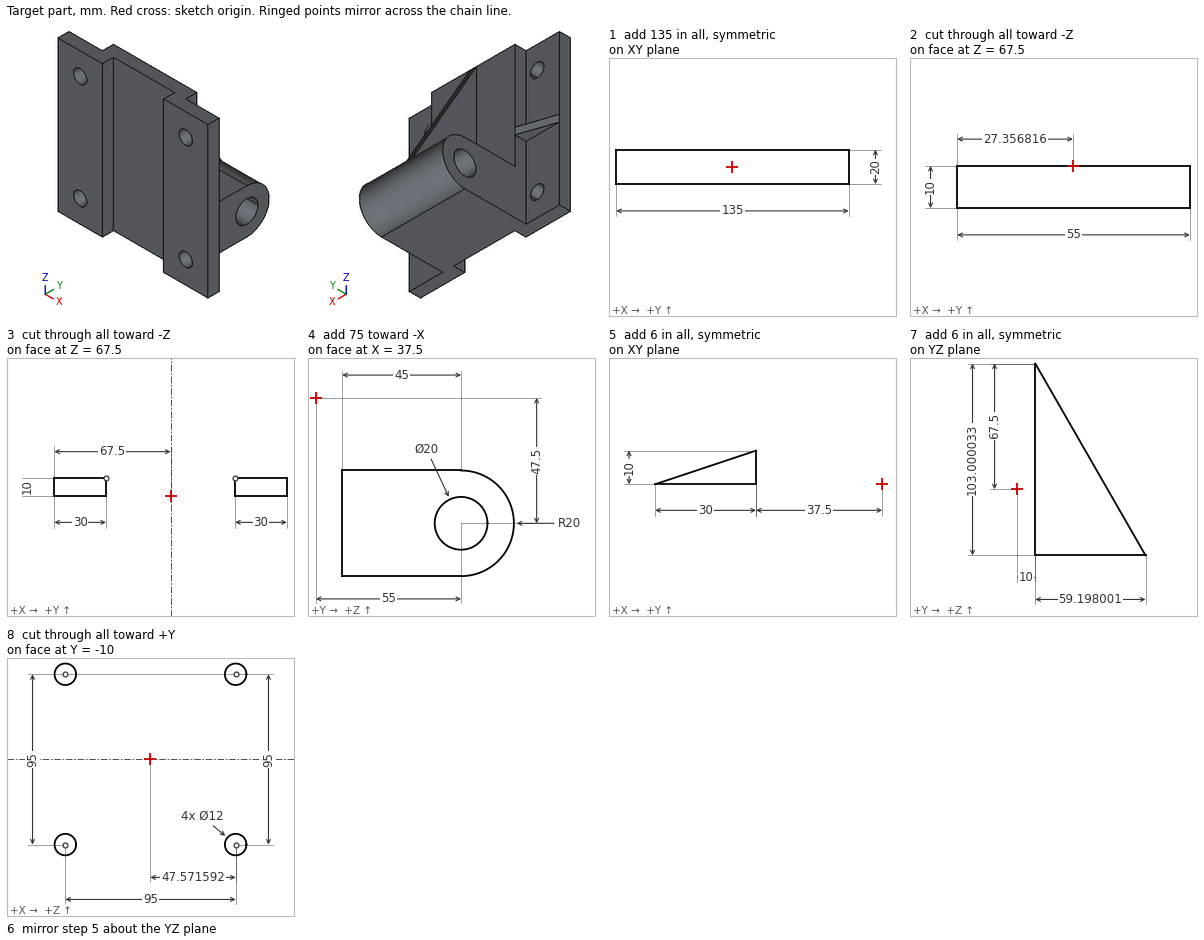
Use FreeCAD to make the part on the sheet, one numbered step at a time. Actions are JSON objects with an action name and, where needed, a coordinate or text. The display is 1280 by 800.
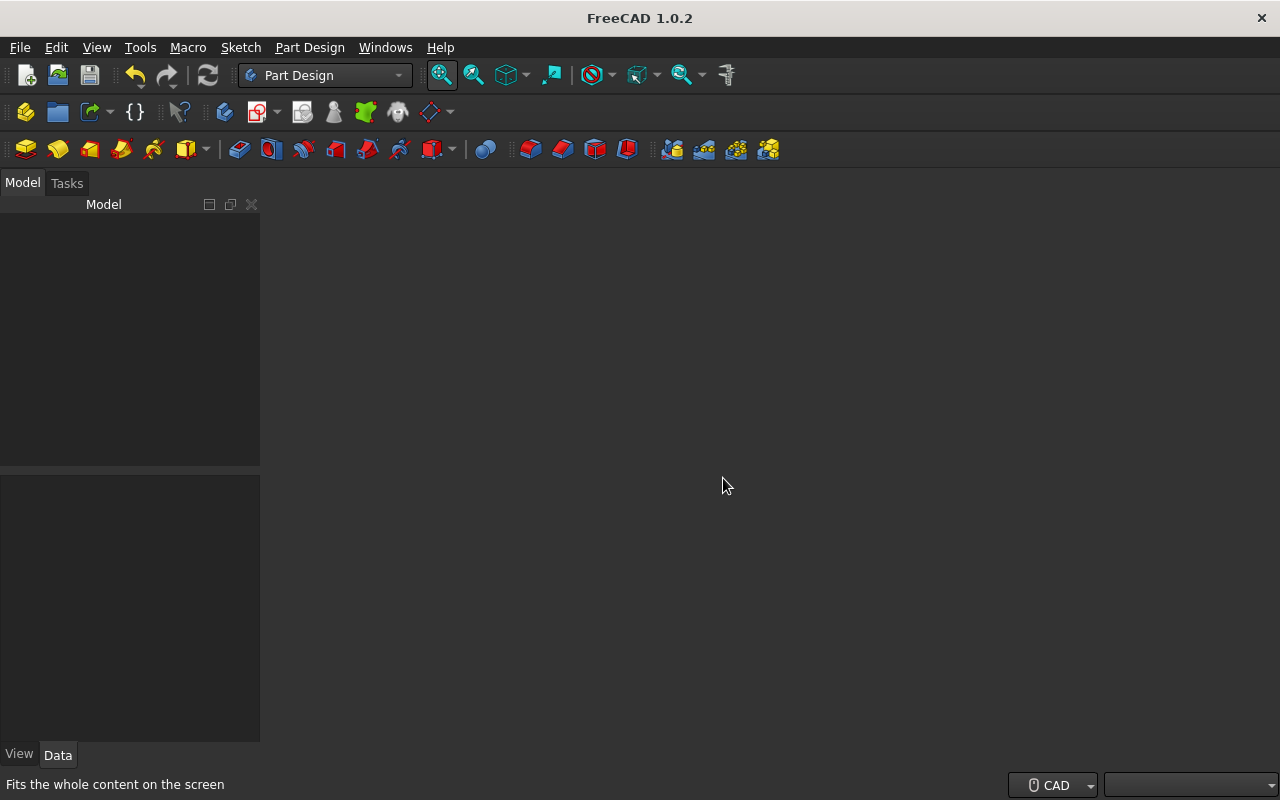
{"action": "left_click", "coordinate": [26, 76]}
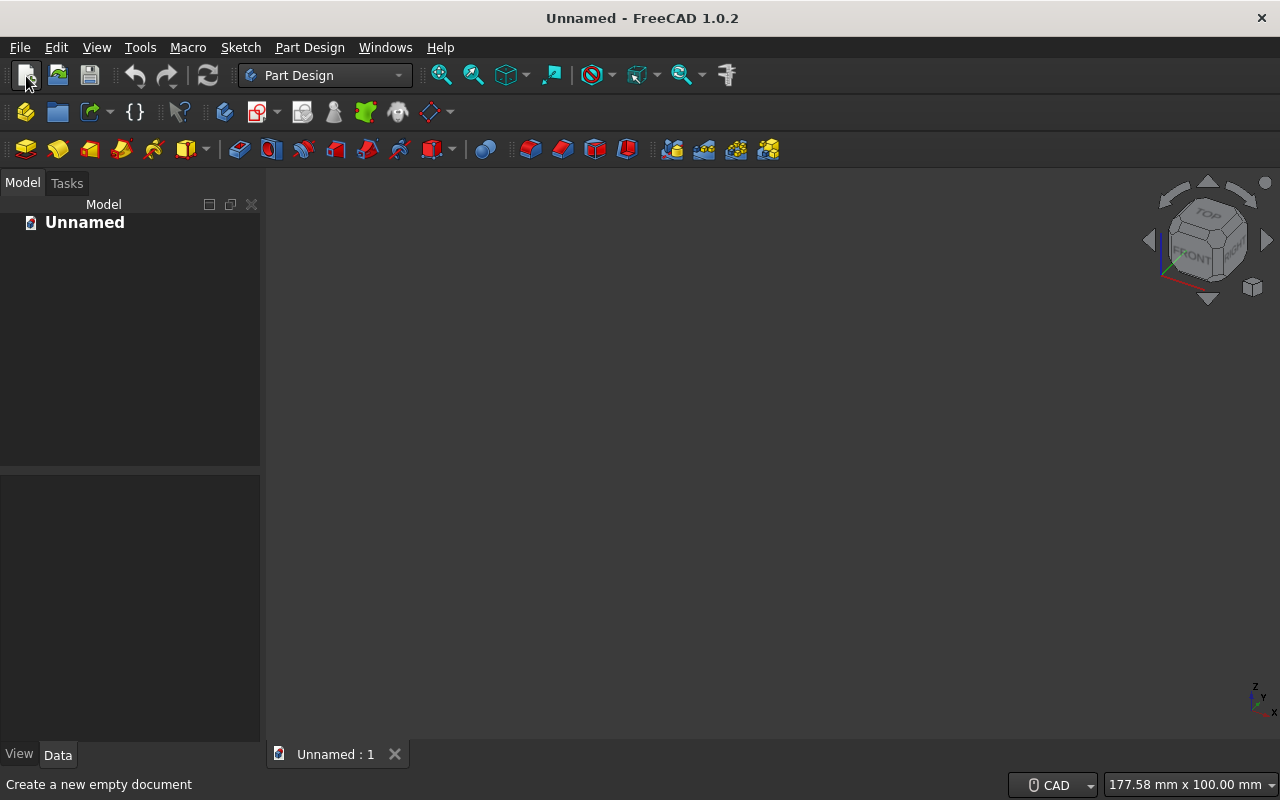
{"action": "left_click", "coordinate": [258, 112]}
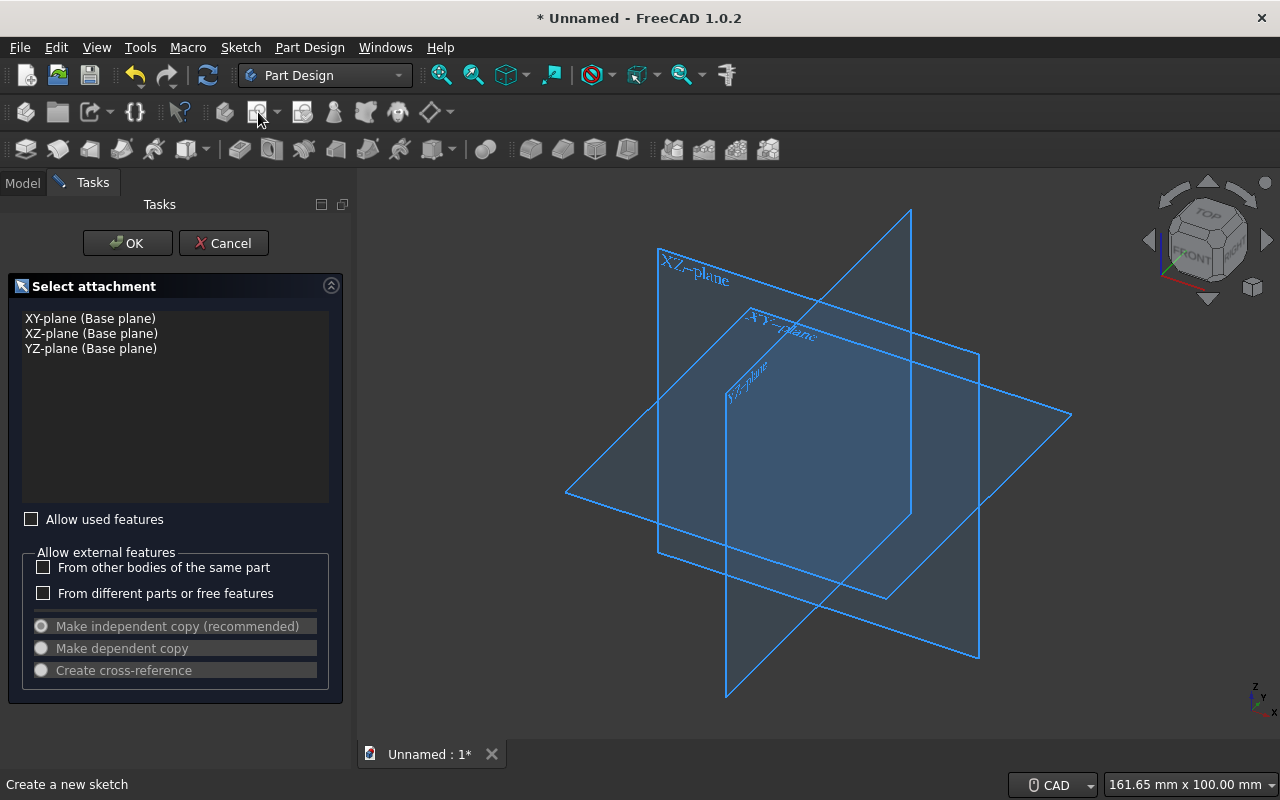
{"action": "left_click", "coordinate": [82, 318]}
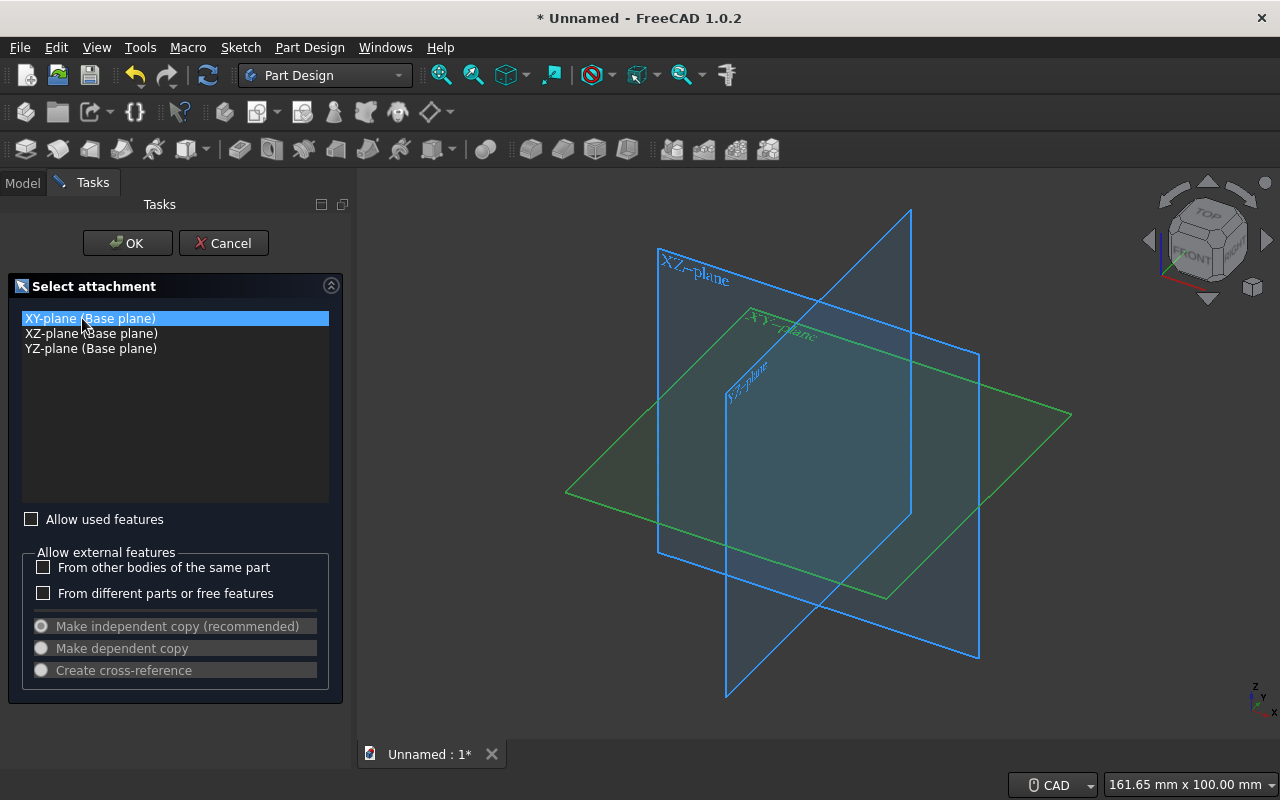
{"action": "left_click", "coordinate": [128, 243]}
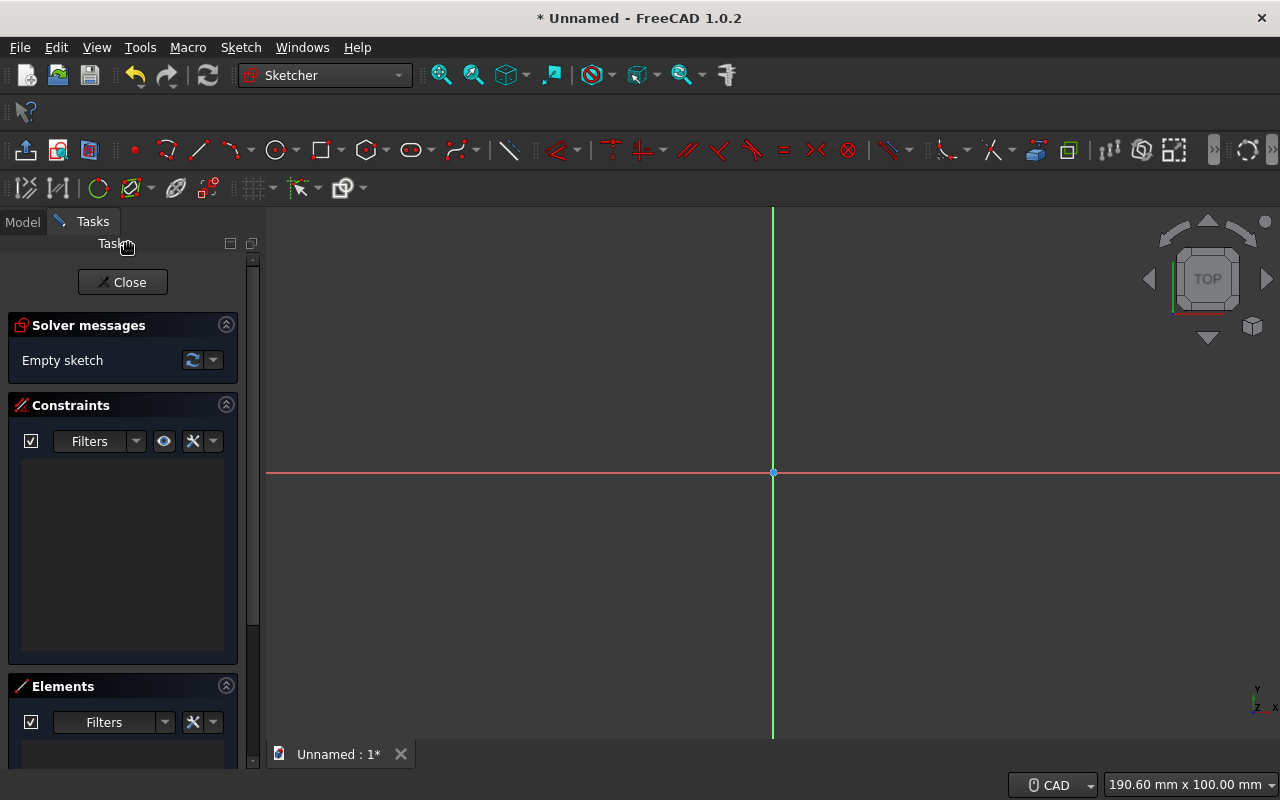
{"action": "scroll", "coordinate": [395, 473], "scroll_direction": "down", "scroll_amount": 1}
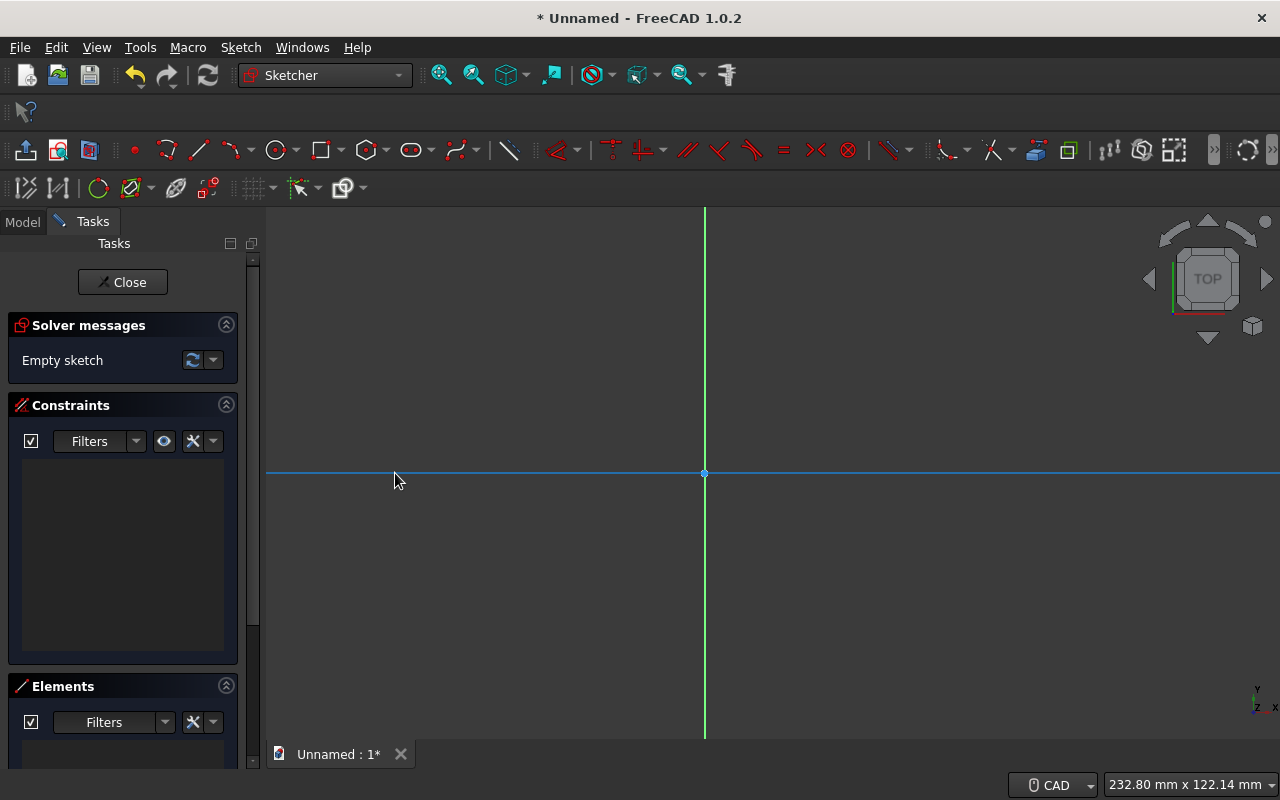
{"action": "key", "text": "g v"}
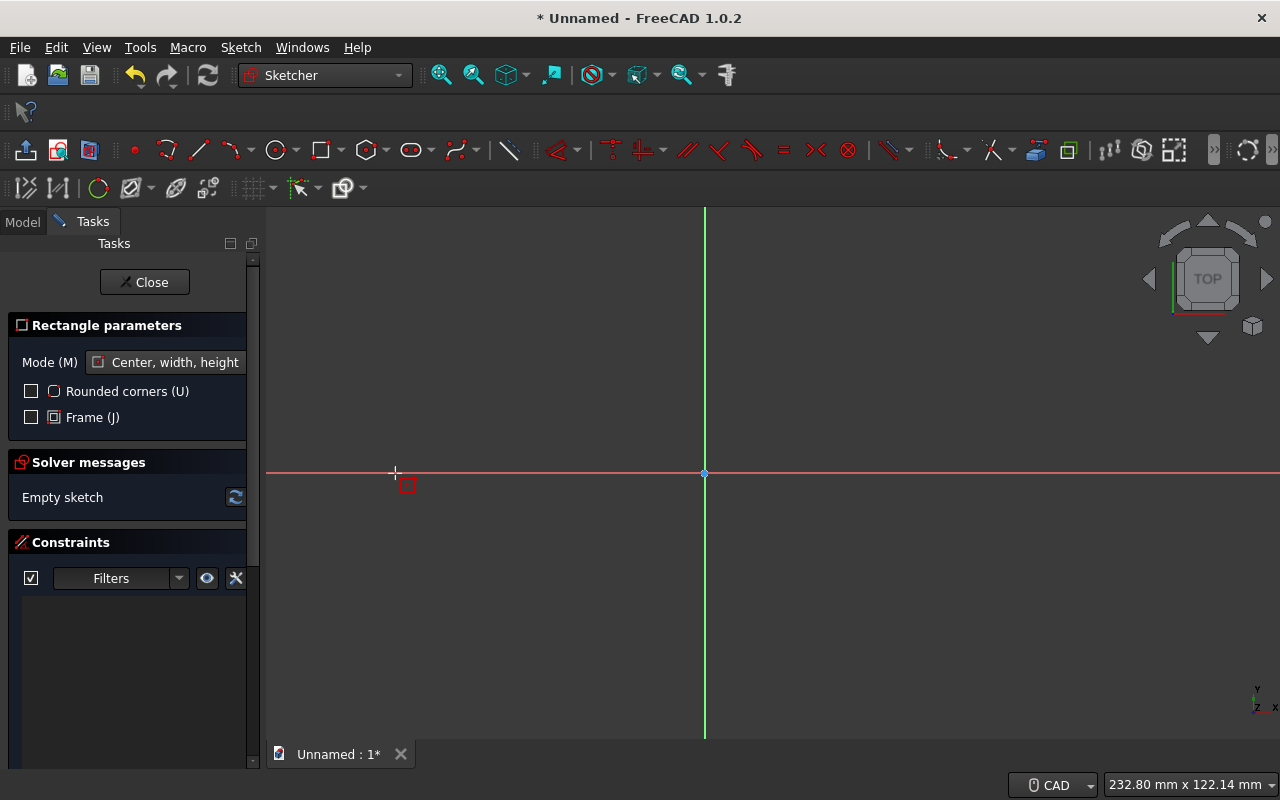
{"action": "left_click", "coordinate": [705, 473]}
{"action": "left_click", "coordinate": [999, 430]}
{"action": "key", "text": "Escape"}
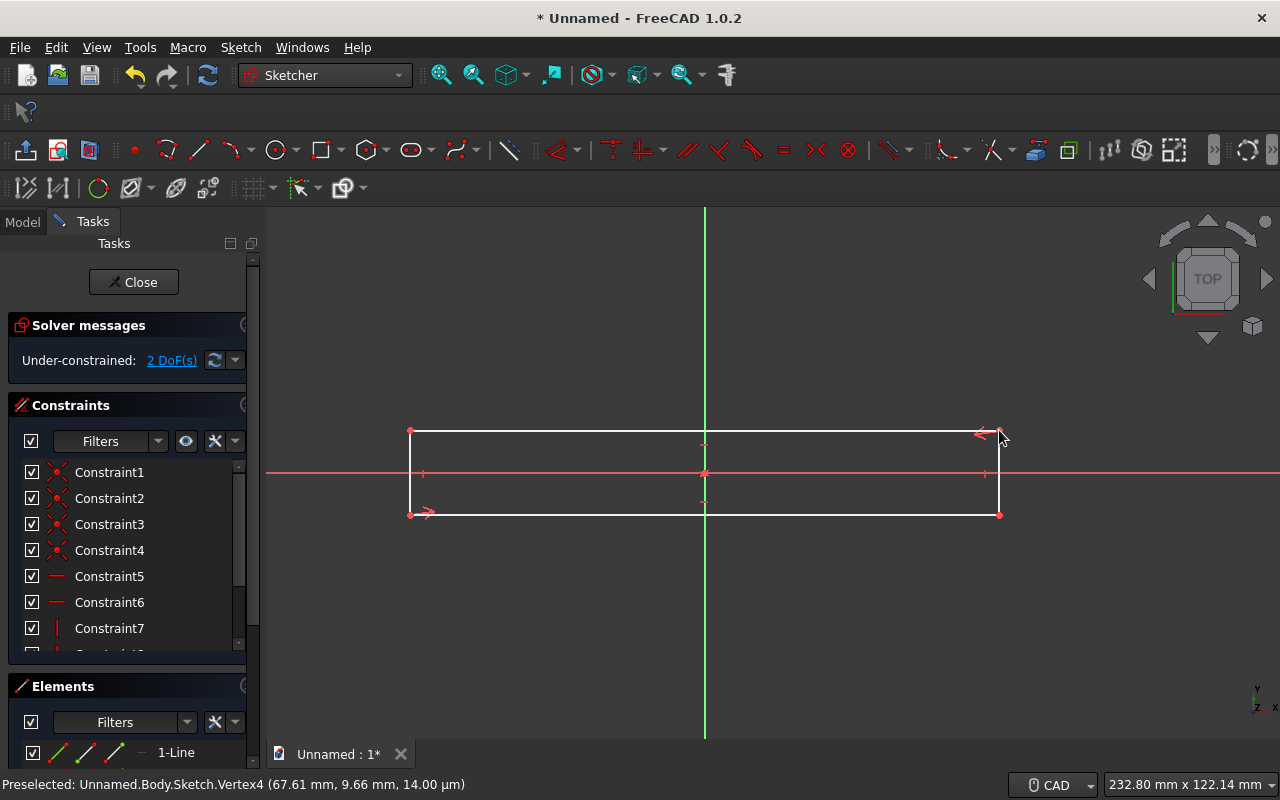
{"action": "left_click", "coordinate": [556, 150]}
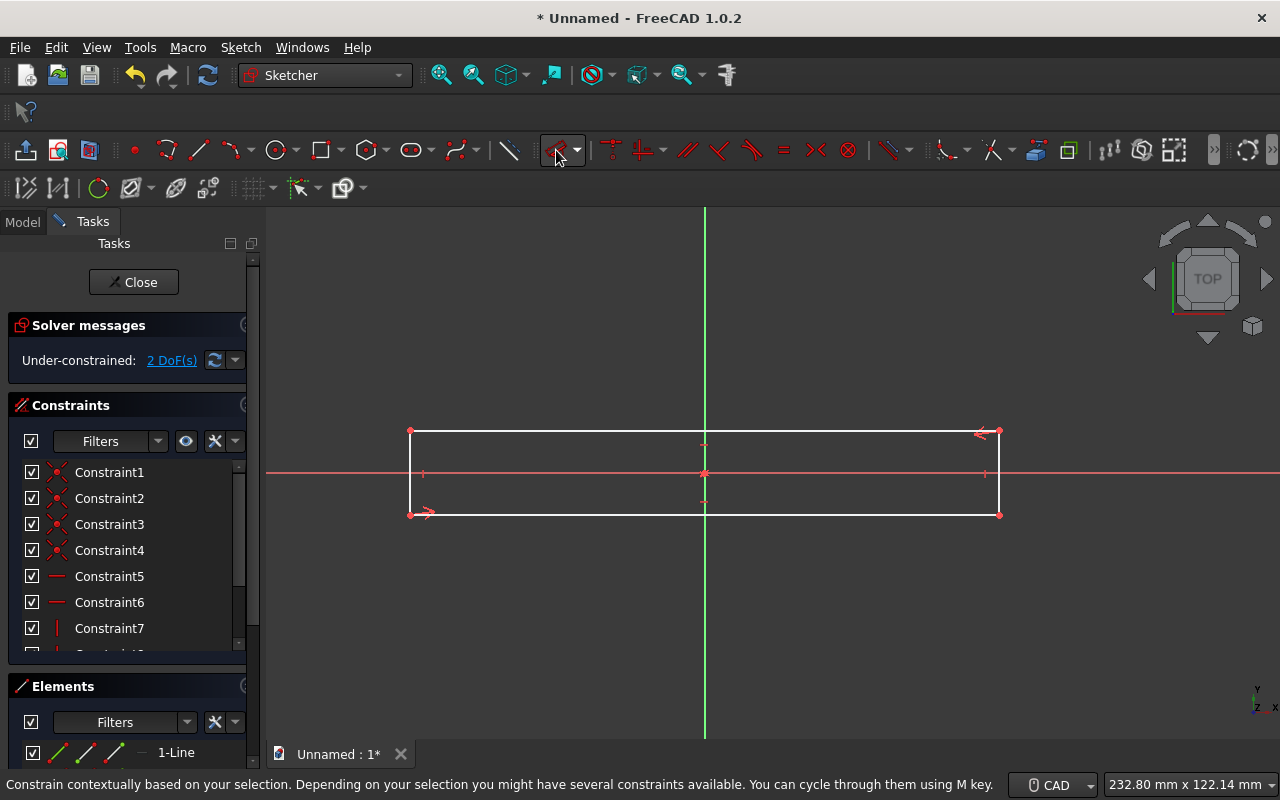
{"action": "left_click", "coordinate": [999, 490]}
{"action": "left_click", "coordinate": [1033, 454]}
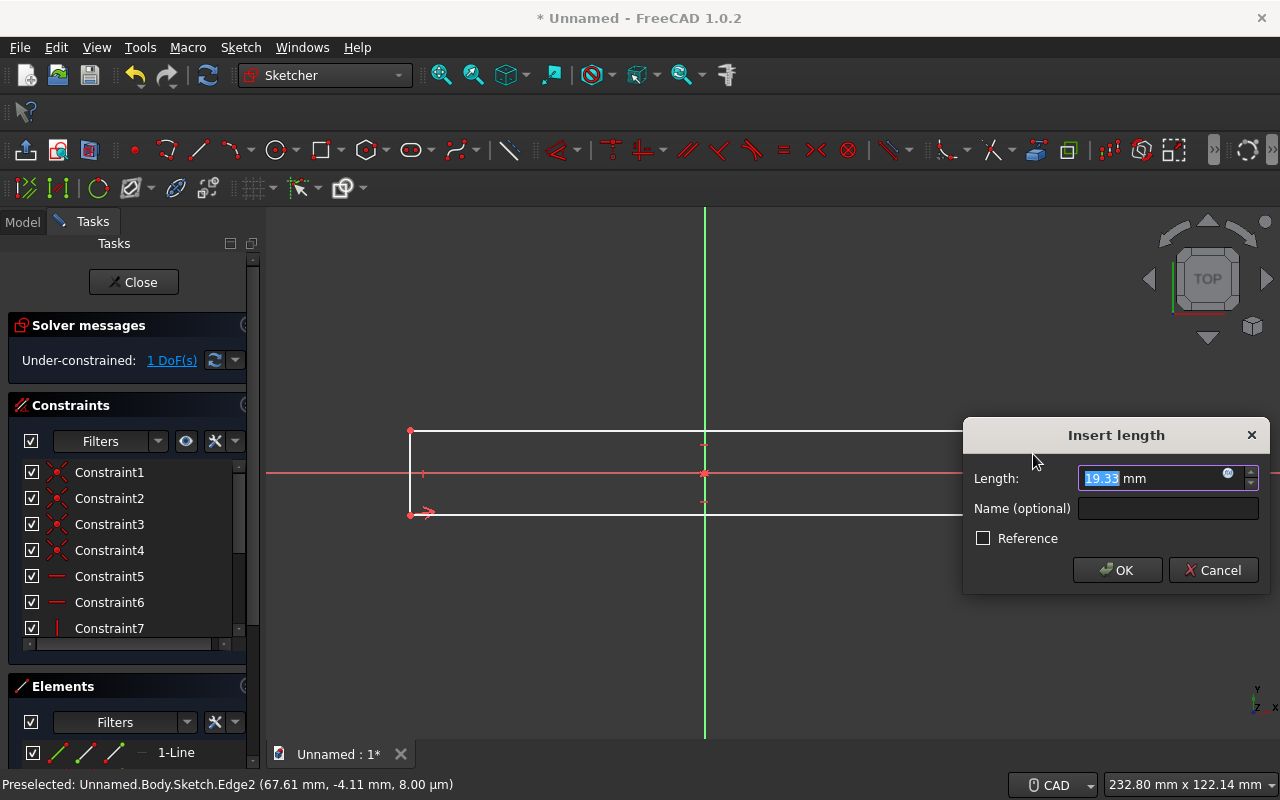
{"action": "type", "text": "20"}
{"action": "key", "text": "Return"}